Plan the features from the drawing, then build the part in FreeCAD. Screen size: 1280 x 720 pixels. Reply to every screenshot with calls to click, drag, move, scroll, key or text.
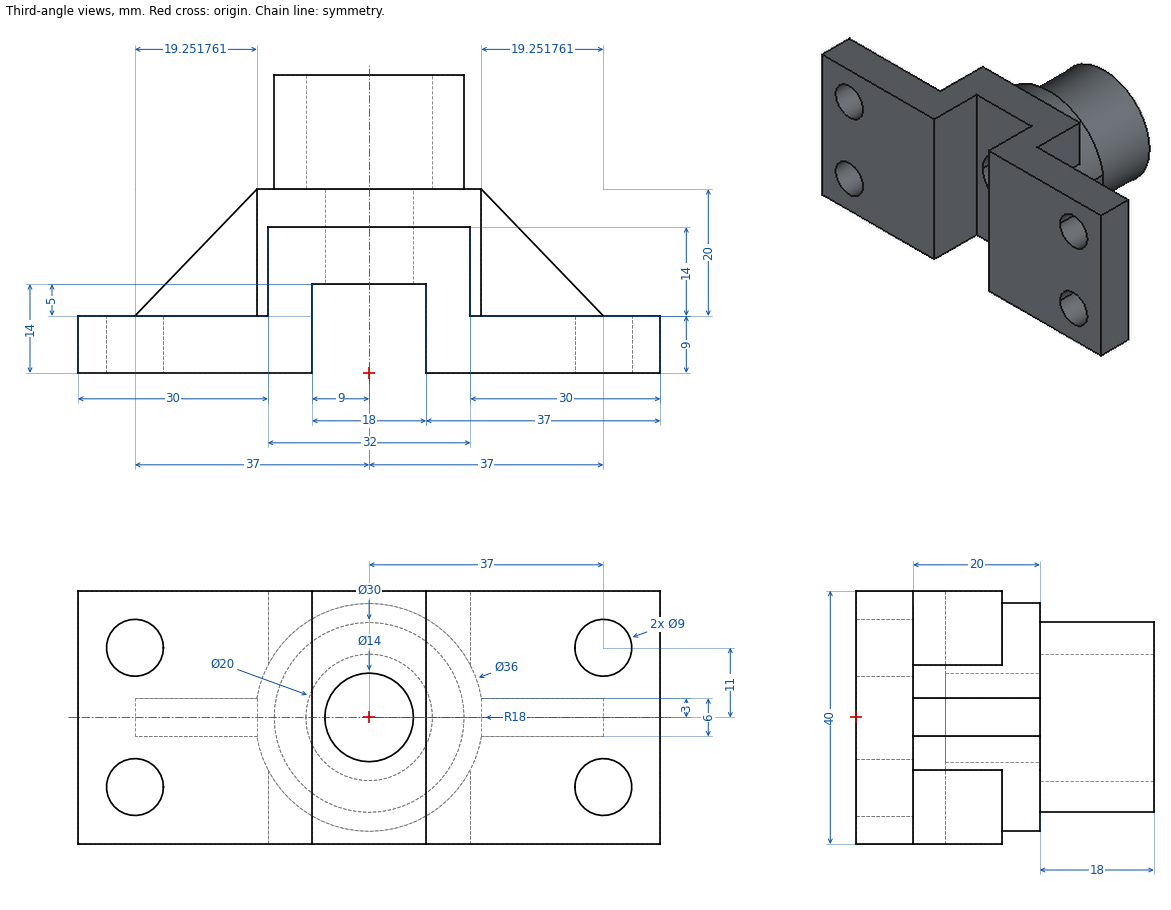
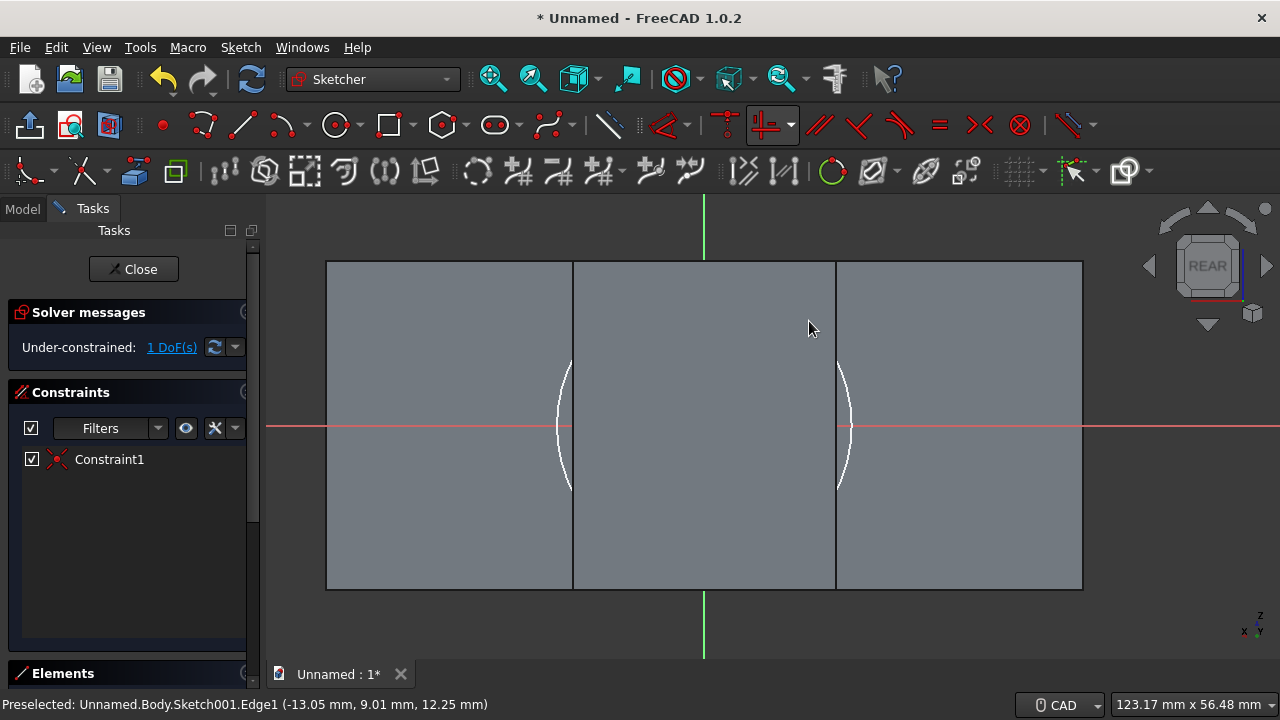
click(664, 126)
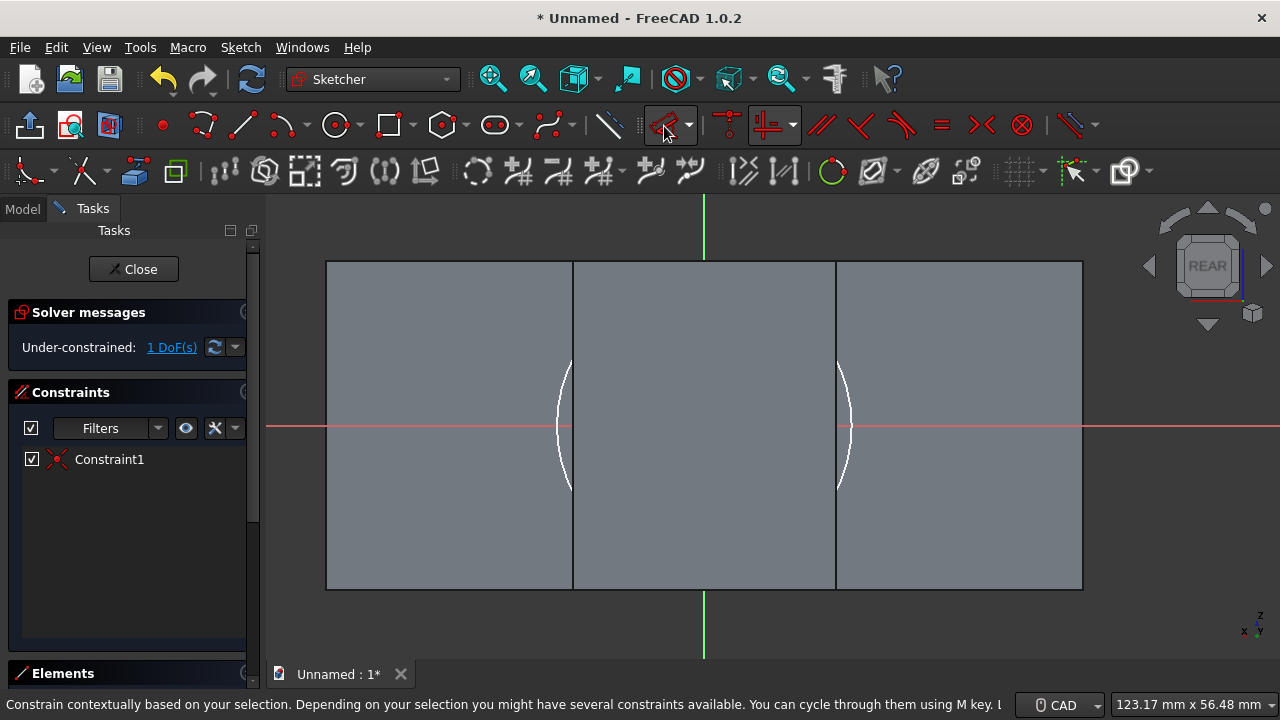
click(808, 321)
click(831, 298)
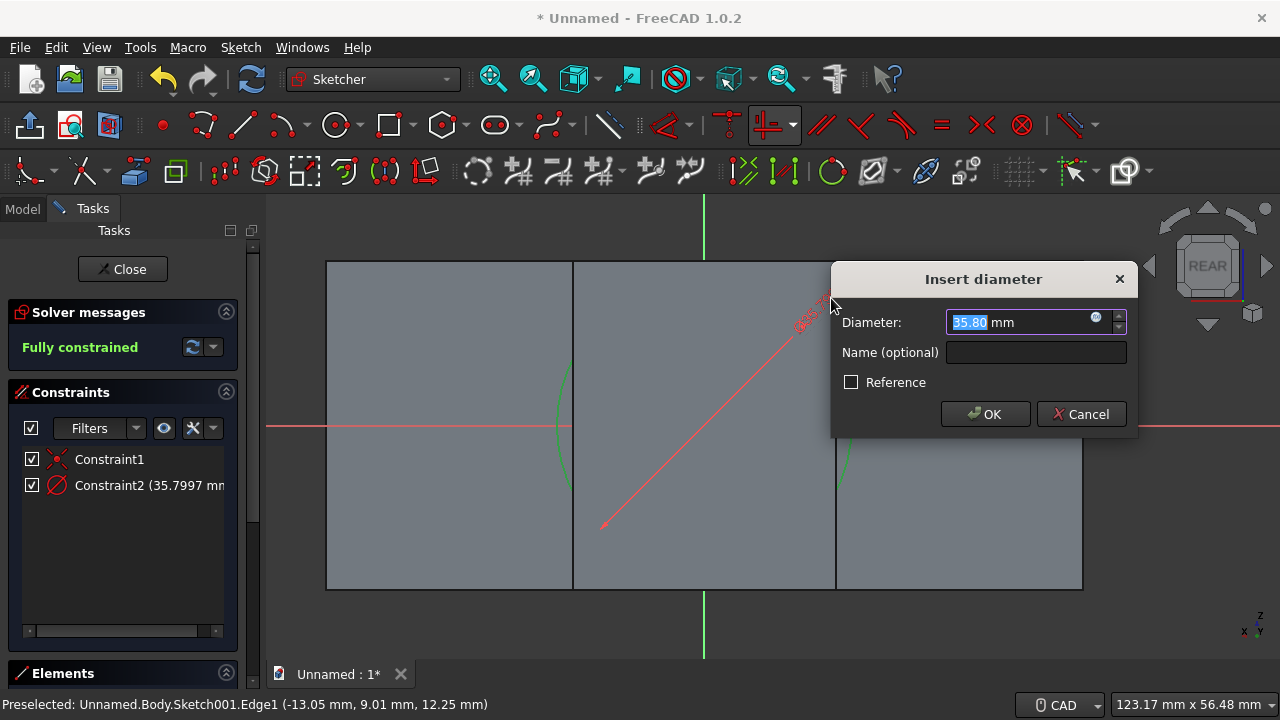
text(36)
key(Return)
key(Escape)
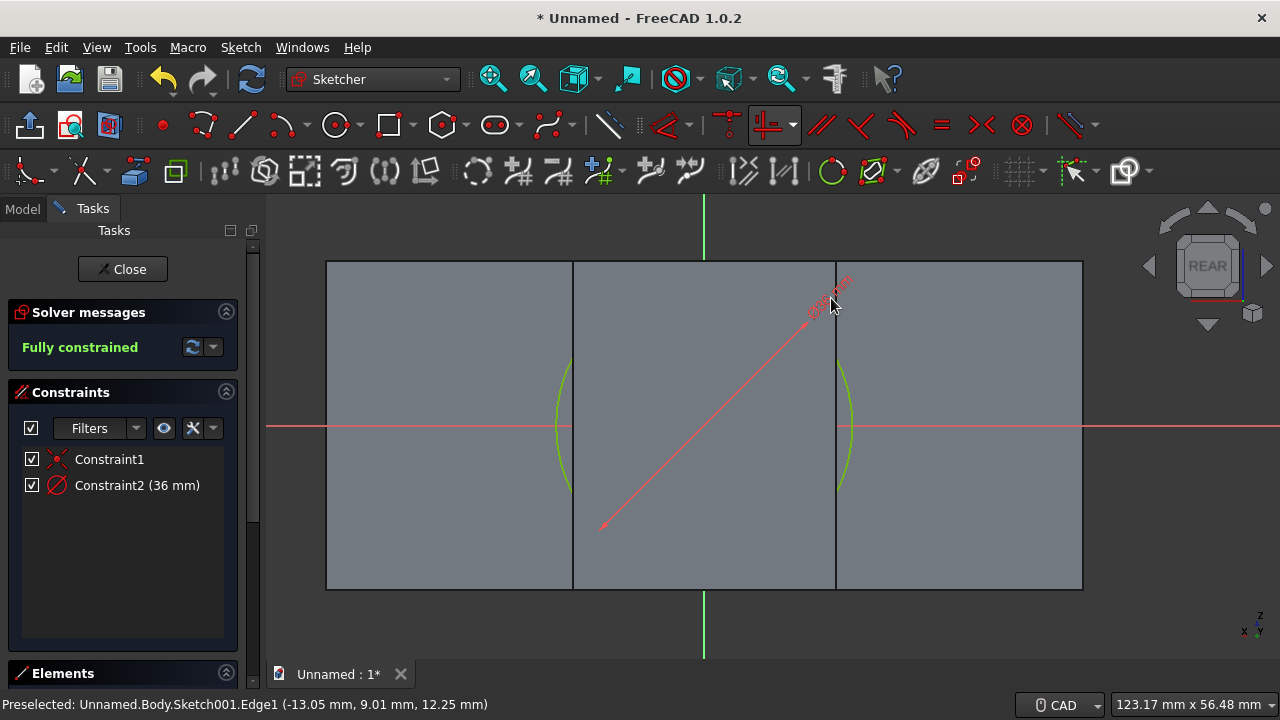
click(123, 269)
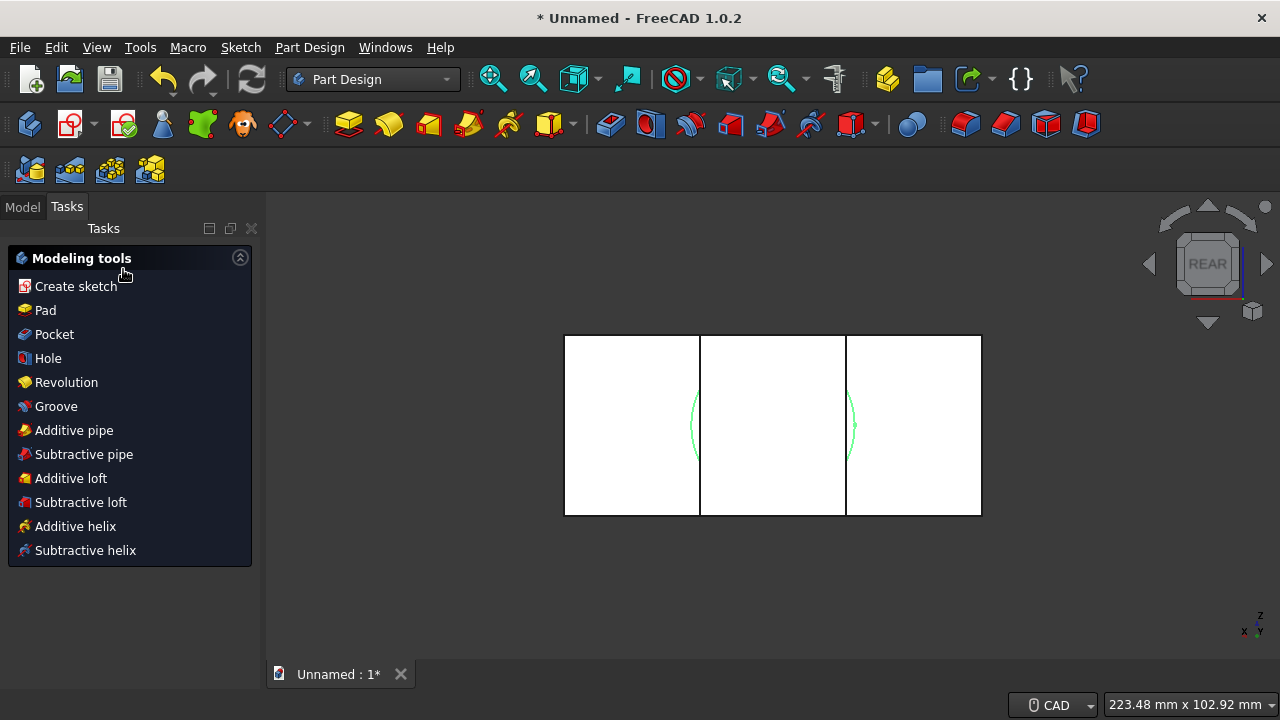
click(350, 124)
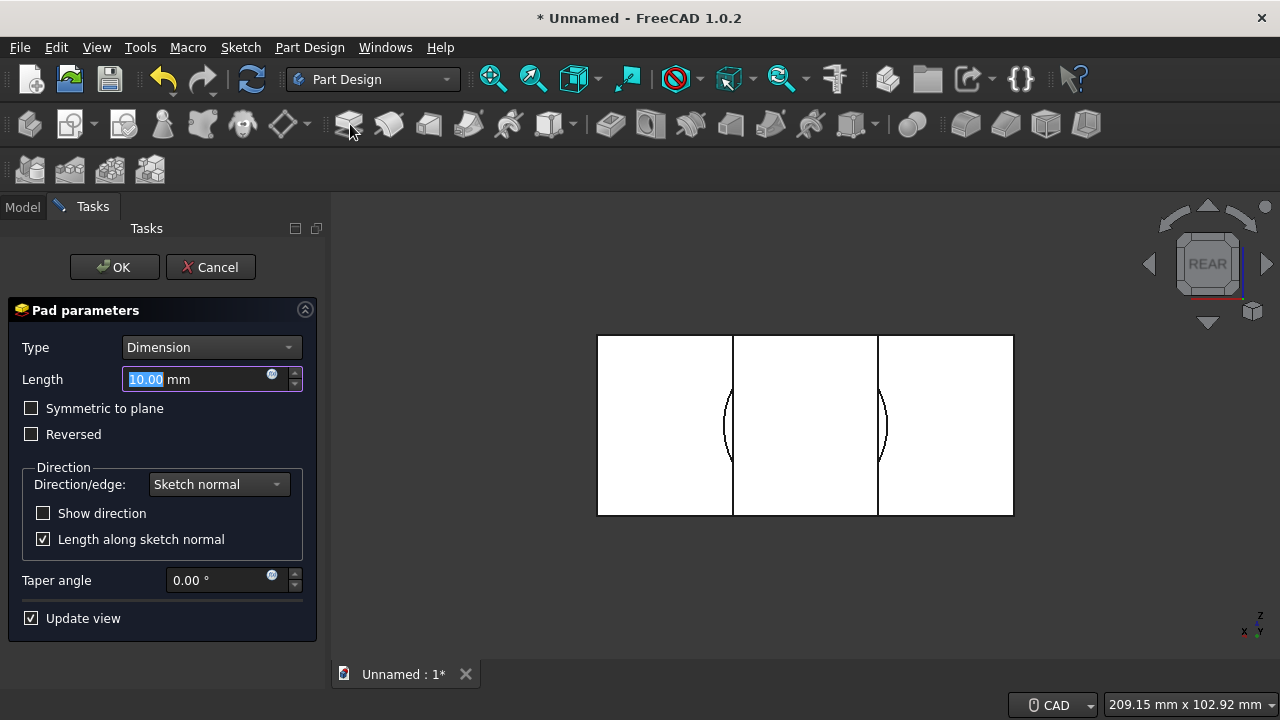
text(20)
key(Tab)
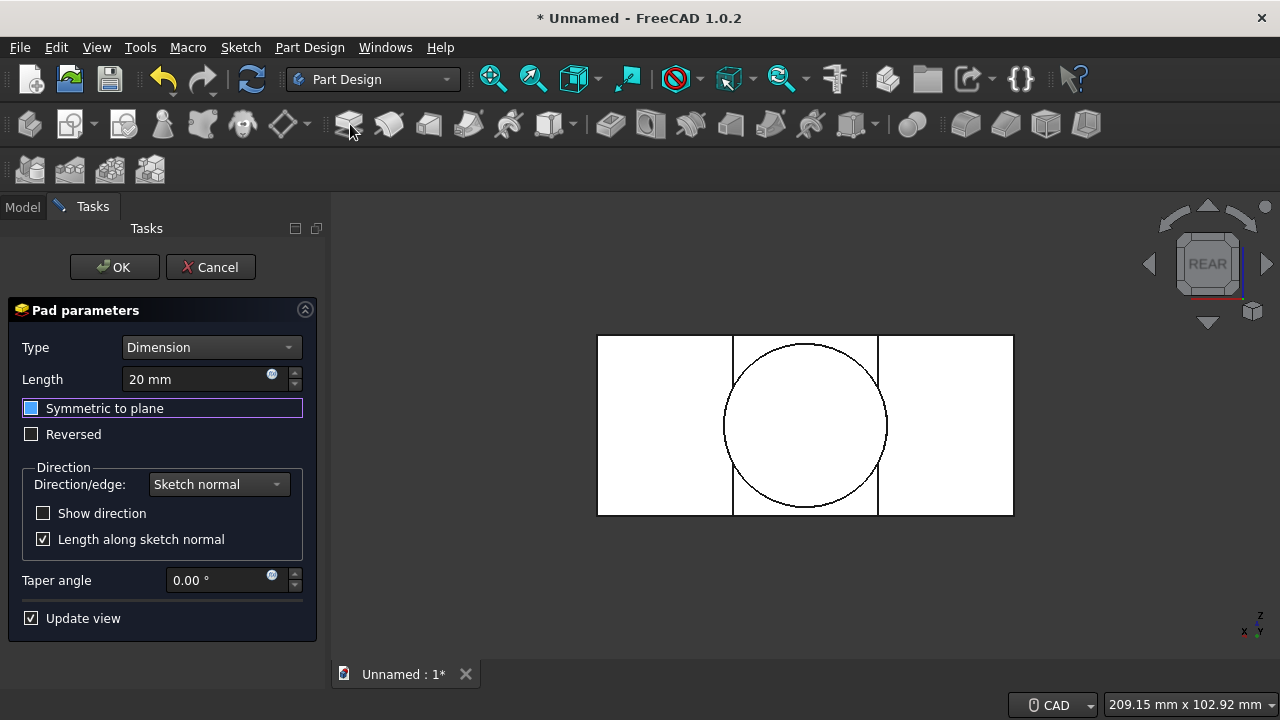
click(115, 267)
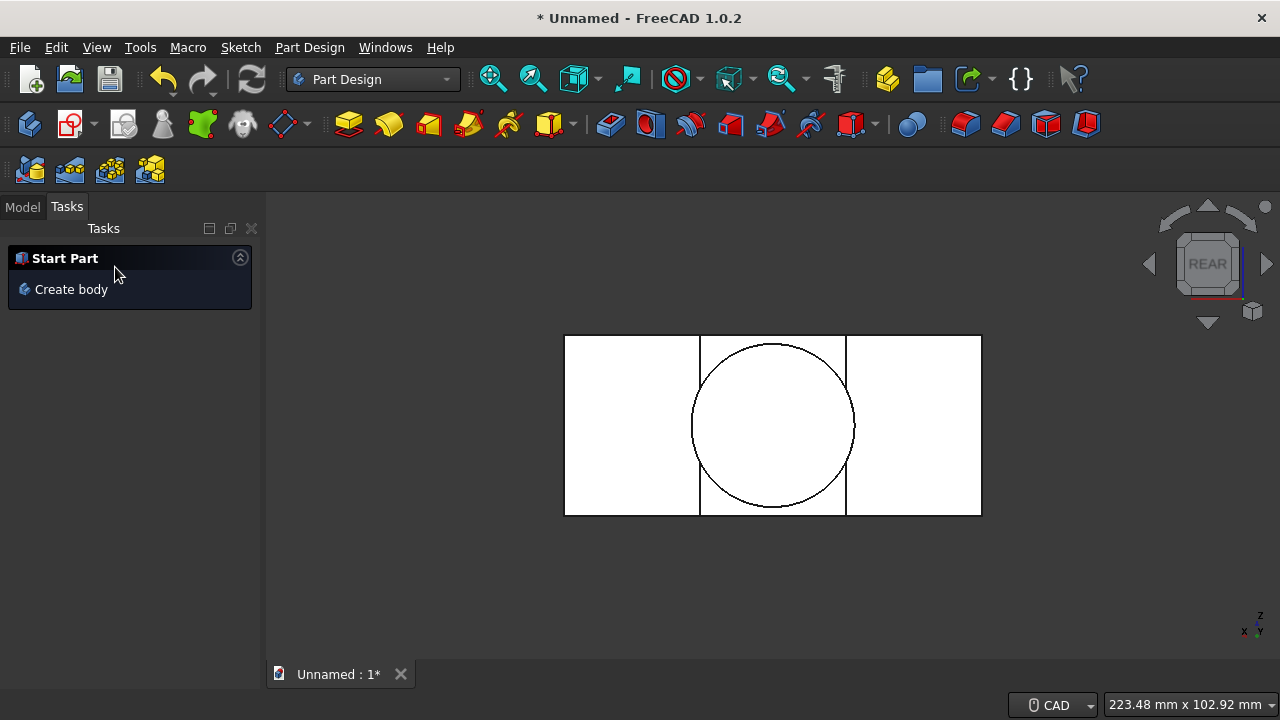
key(v)
key(f)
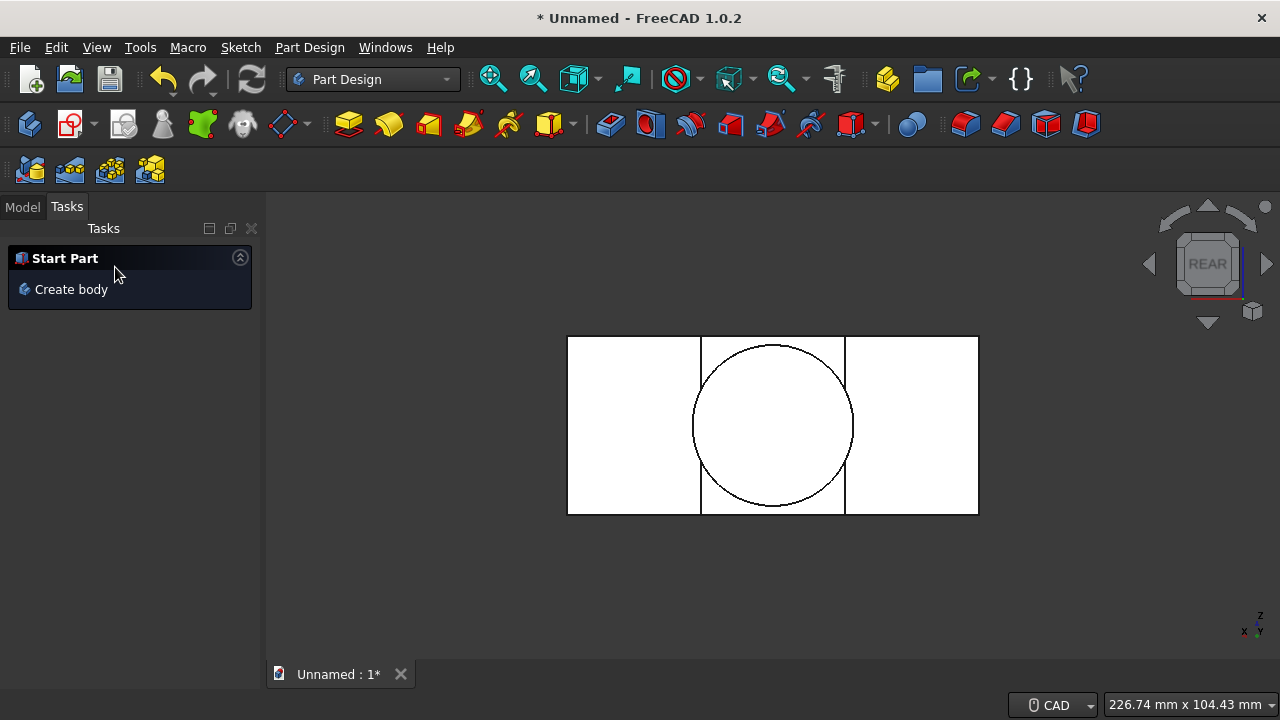
key(0)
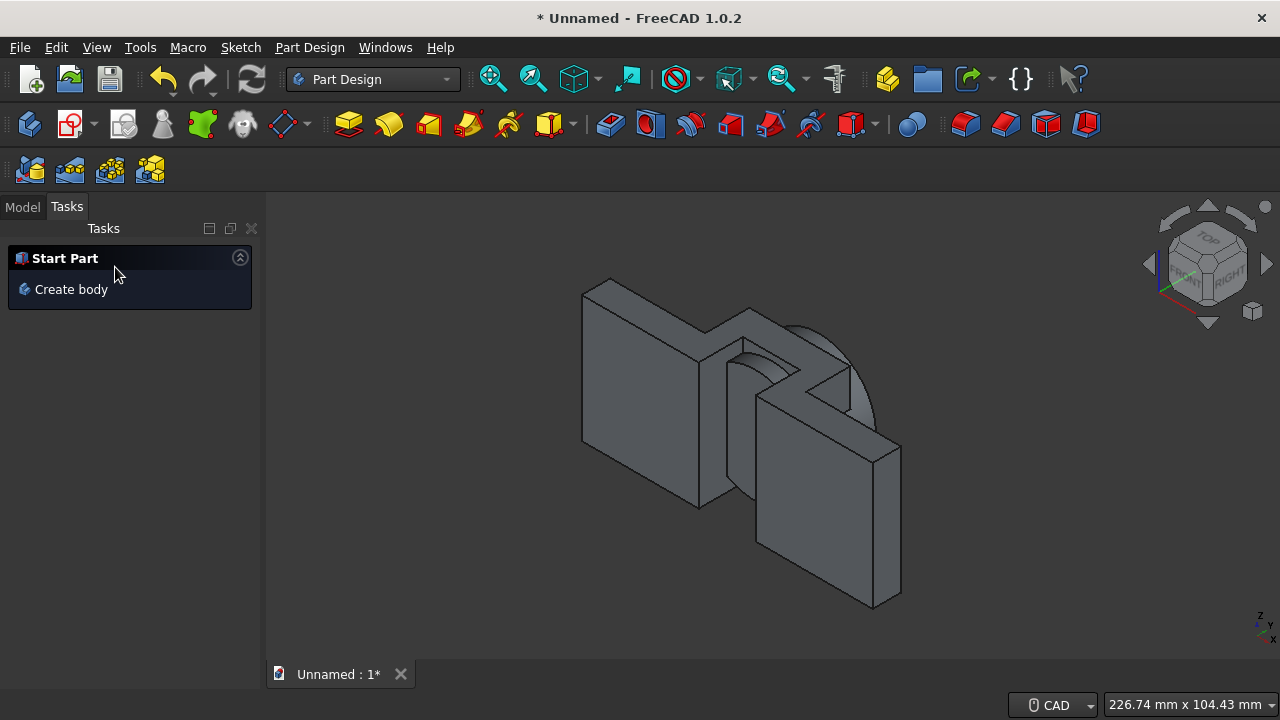
click(701, 345)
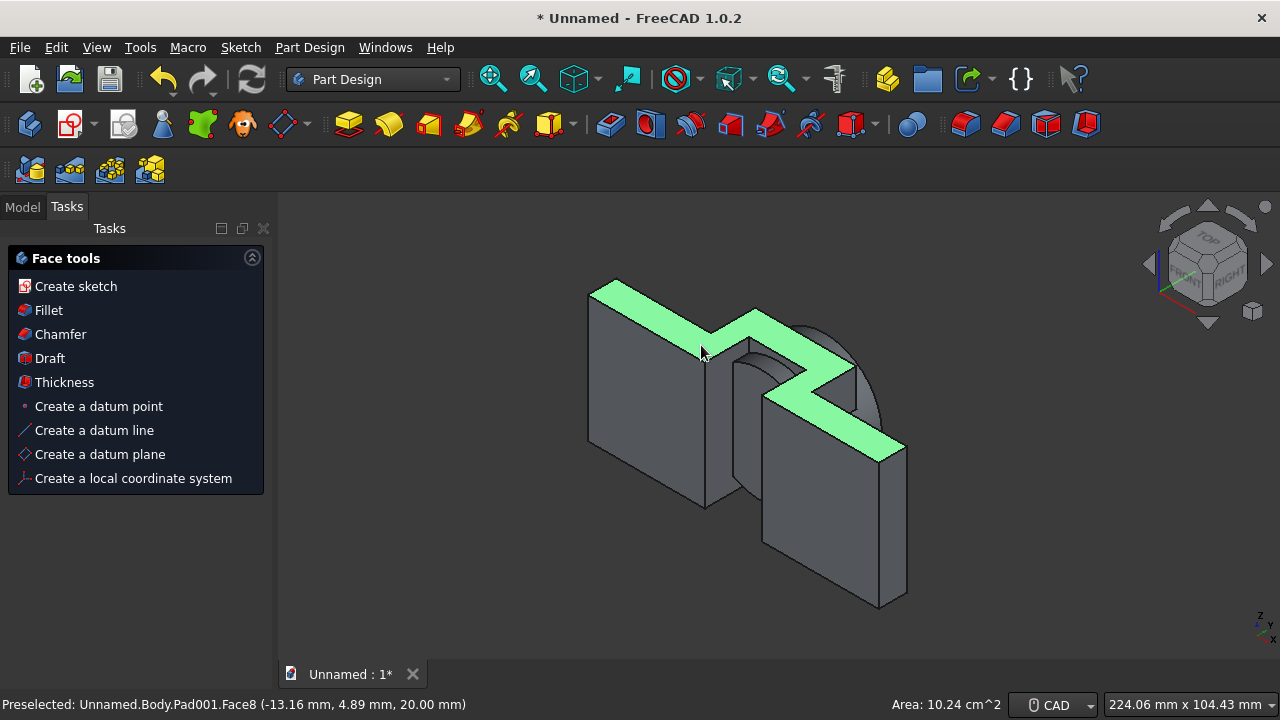
click(70, 124)